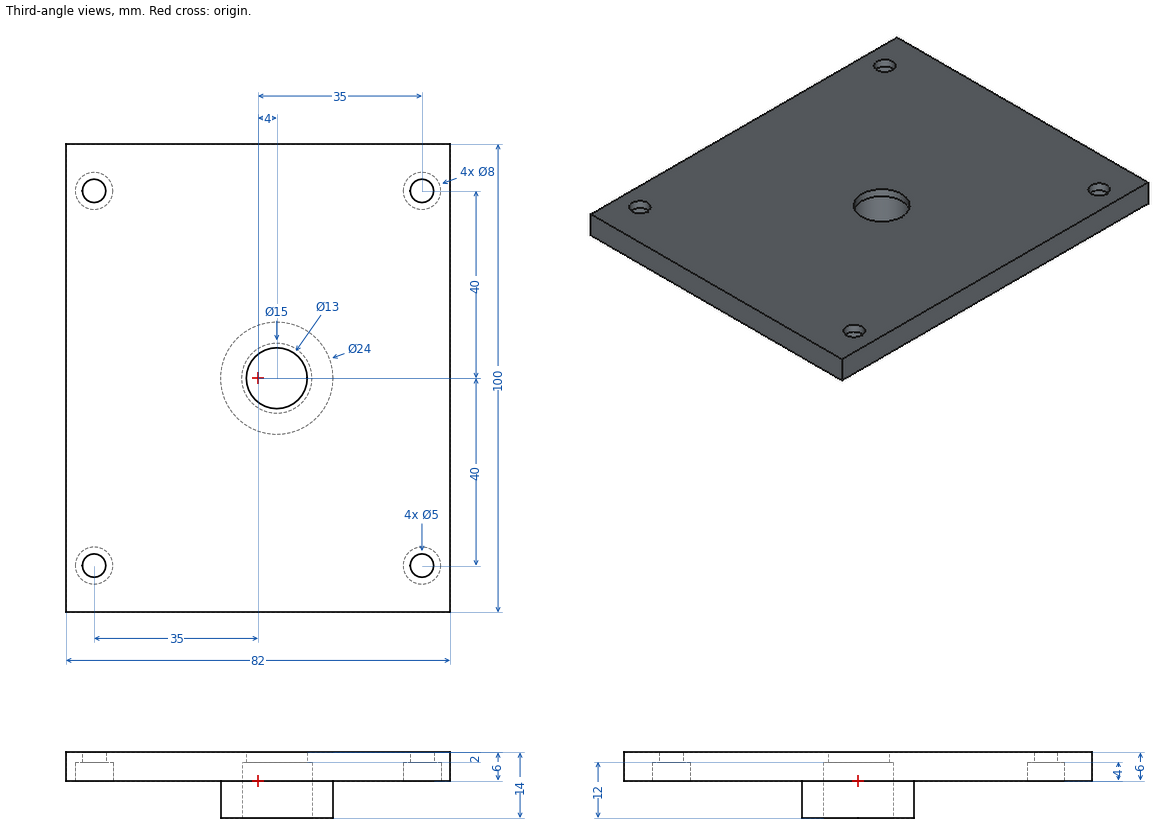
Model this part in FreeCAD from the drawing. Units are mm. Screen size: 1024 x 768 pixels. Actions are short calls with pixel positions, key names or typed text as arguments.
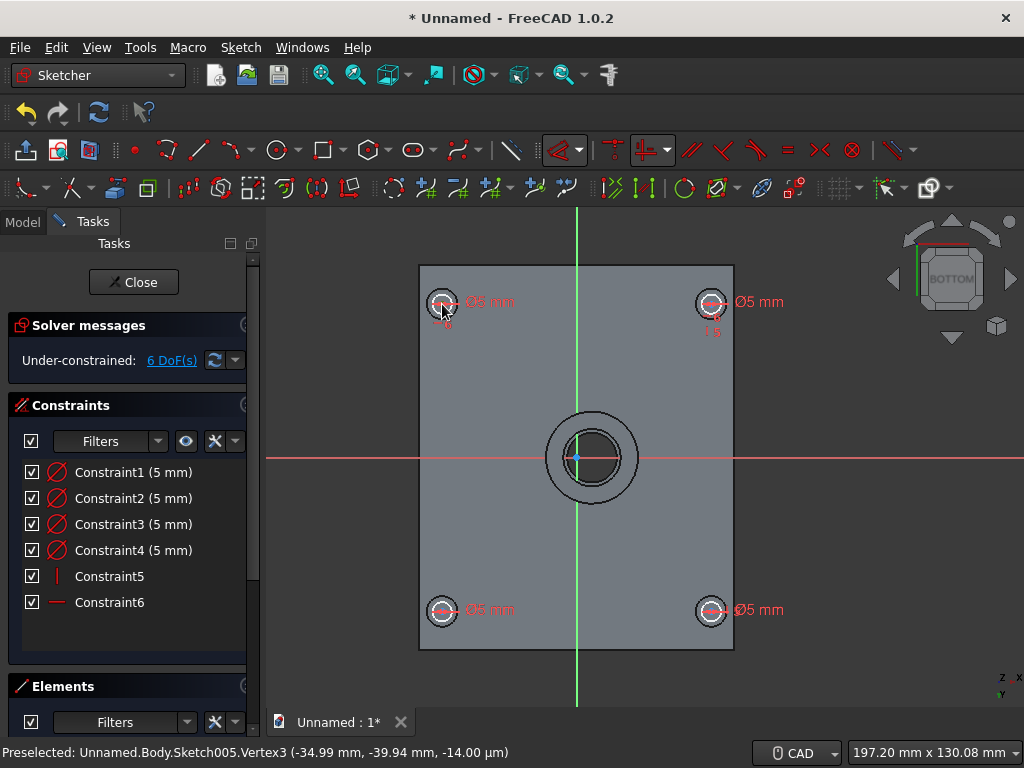
click(442, 612)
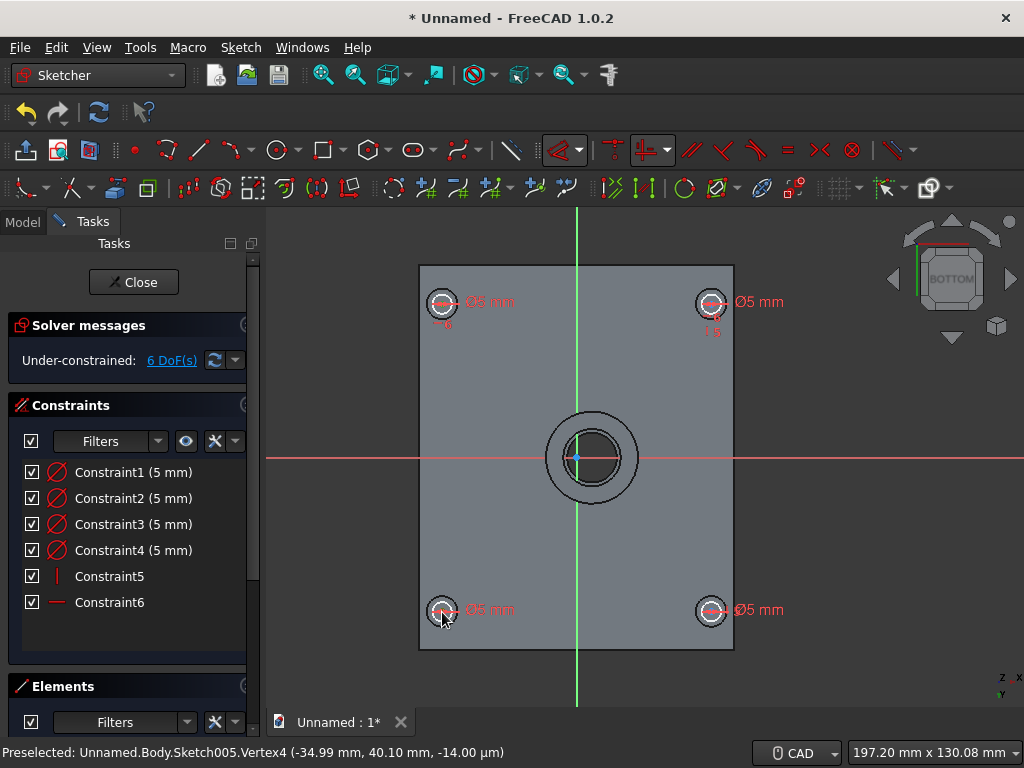
click(670, 150)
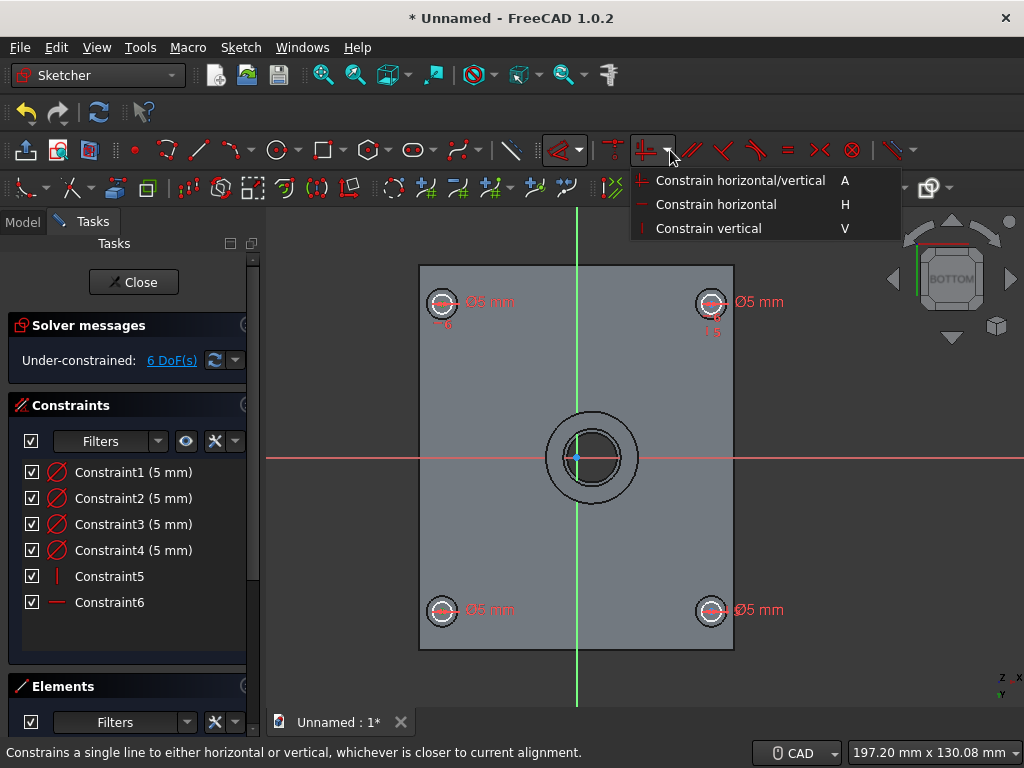
click(766, 228)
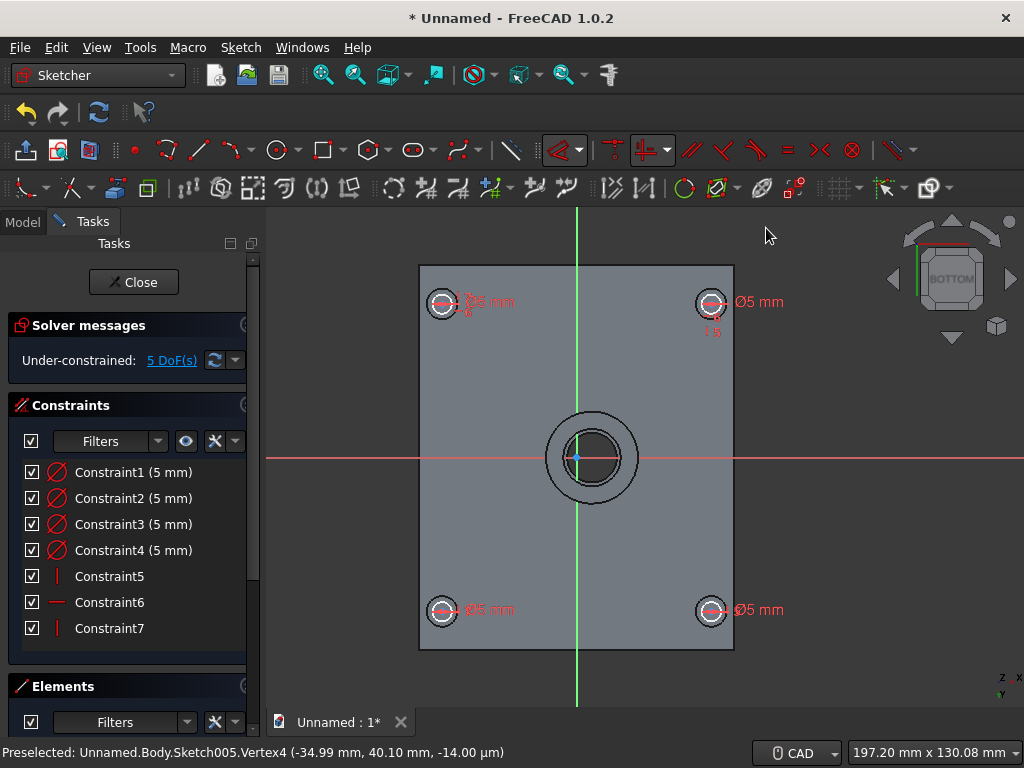
click(711, 612)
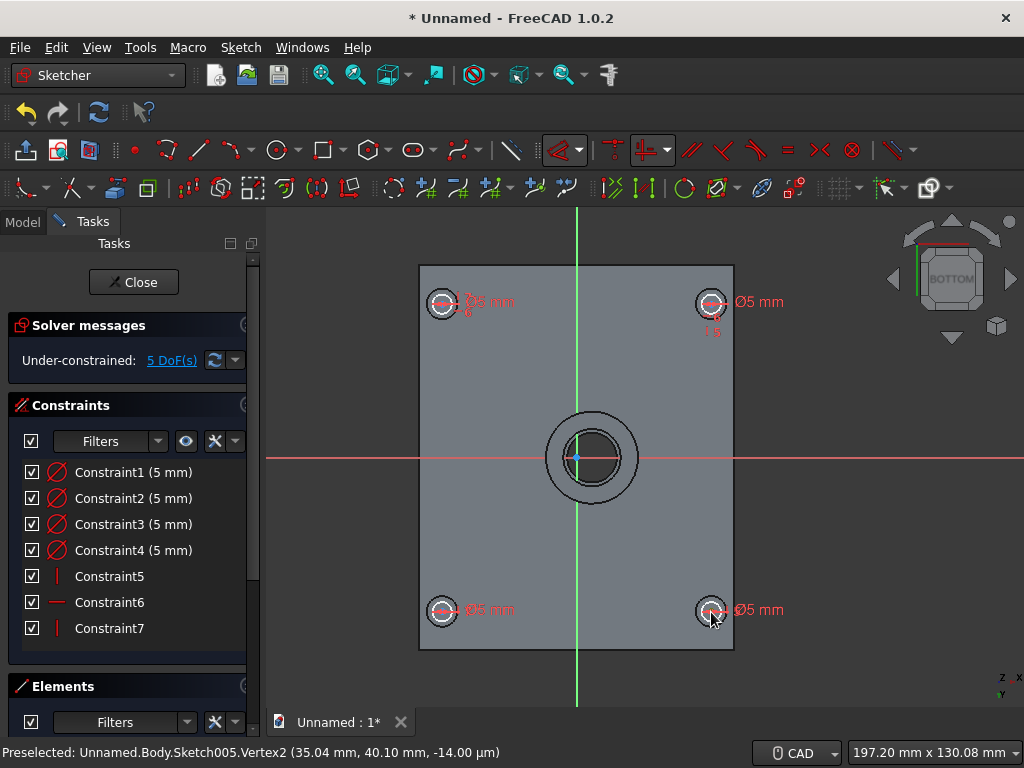
click(442, 612)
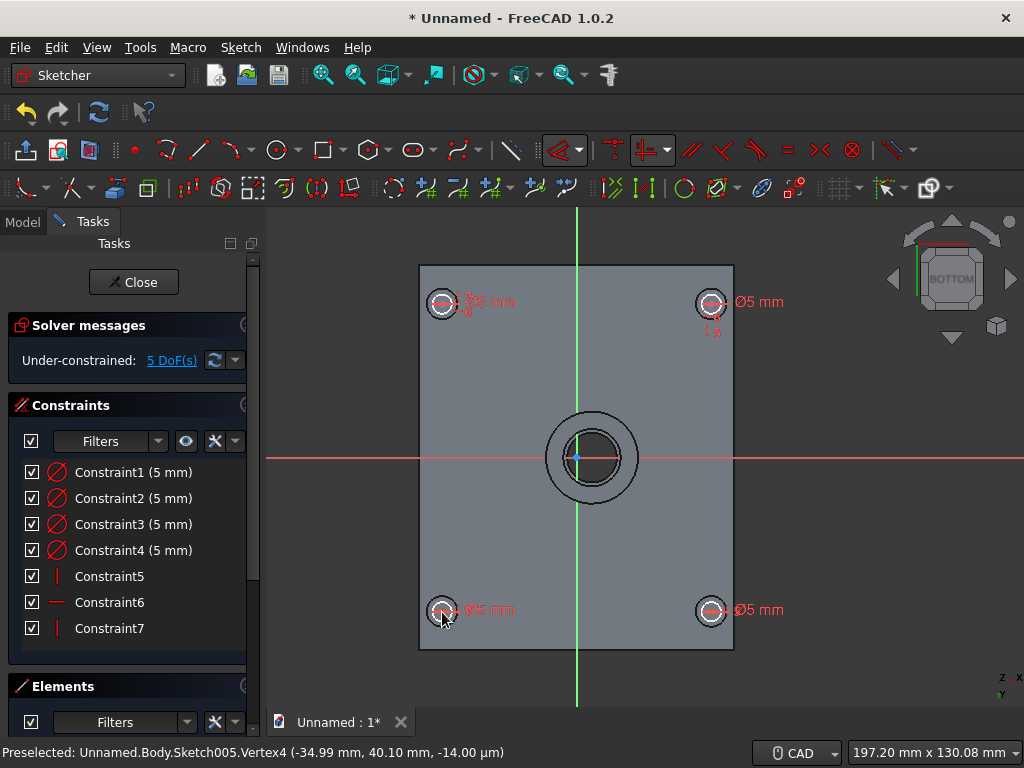
key(h)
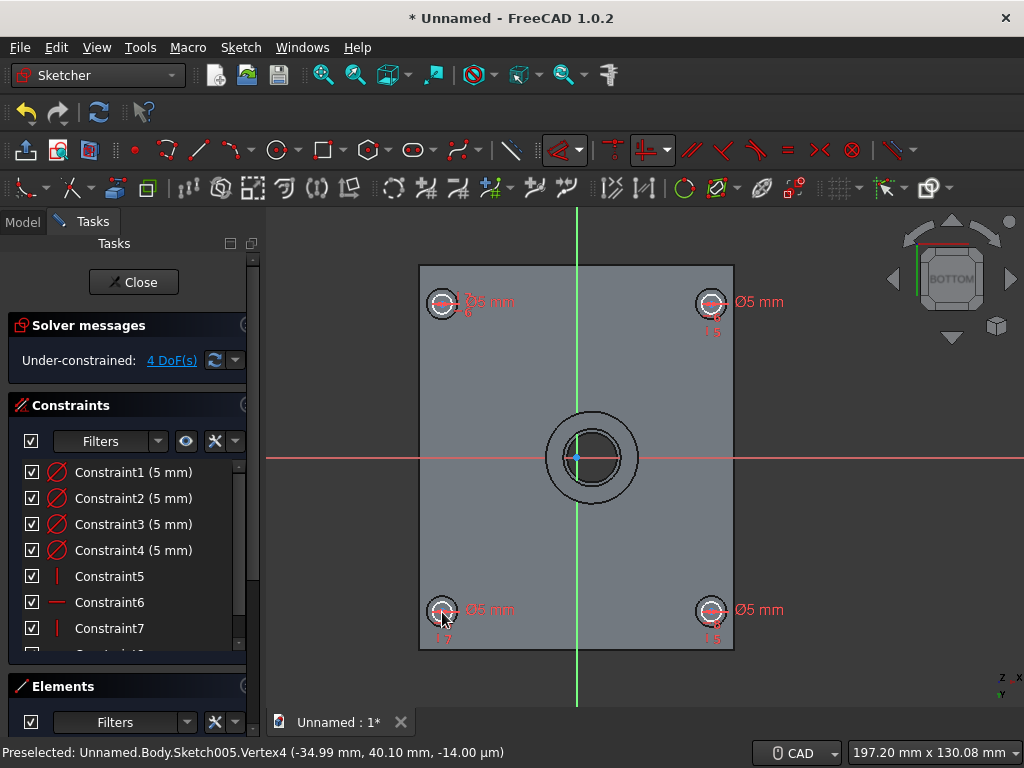
click(711, 304)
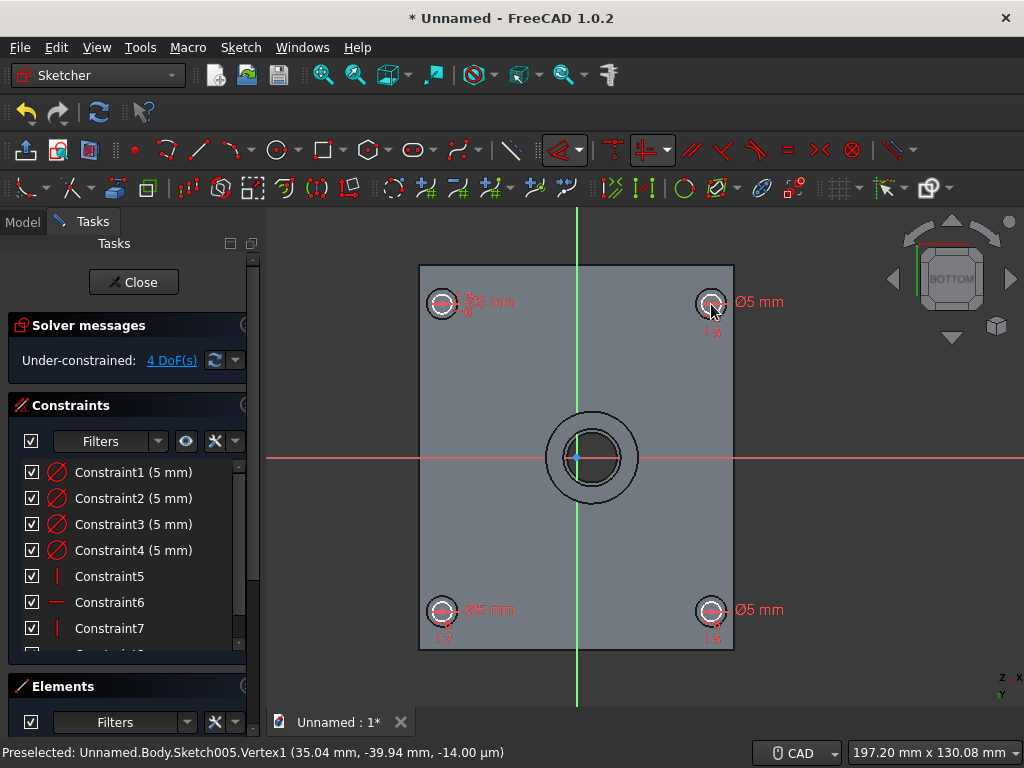
click(582, 150)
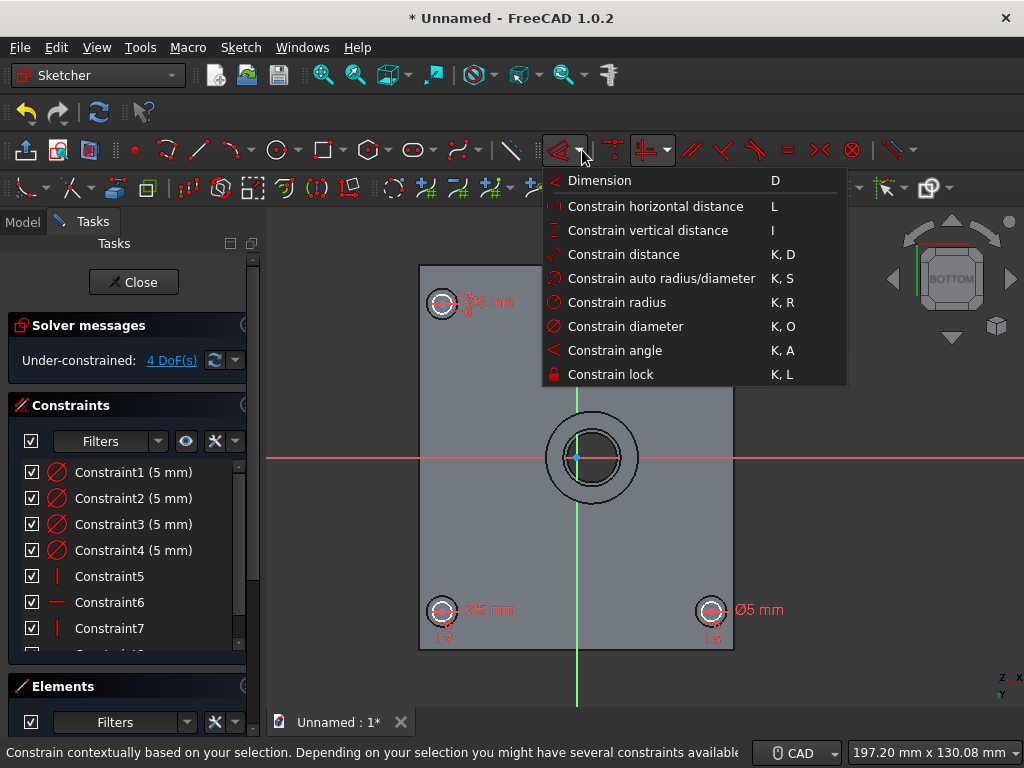
click(695, 206)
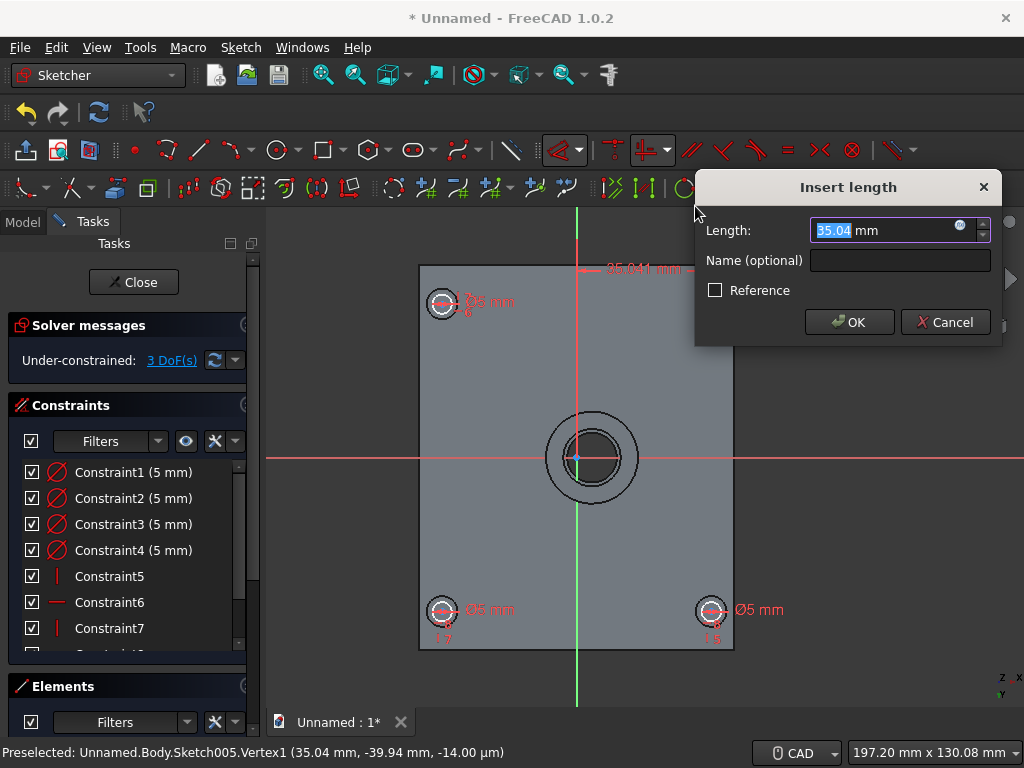
text(35)
key(Return)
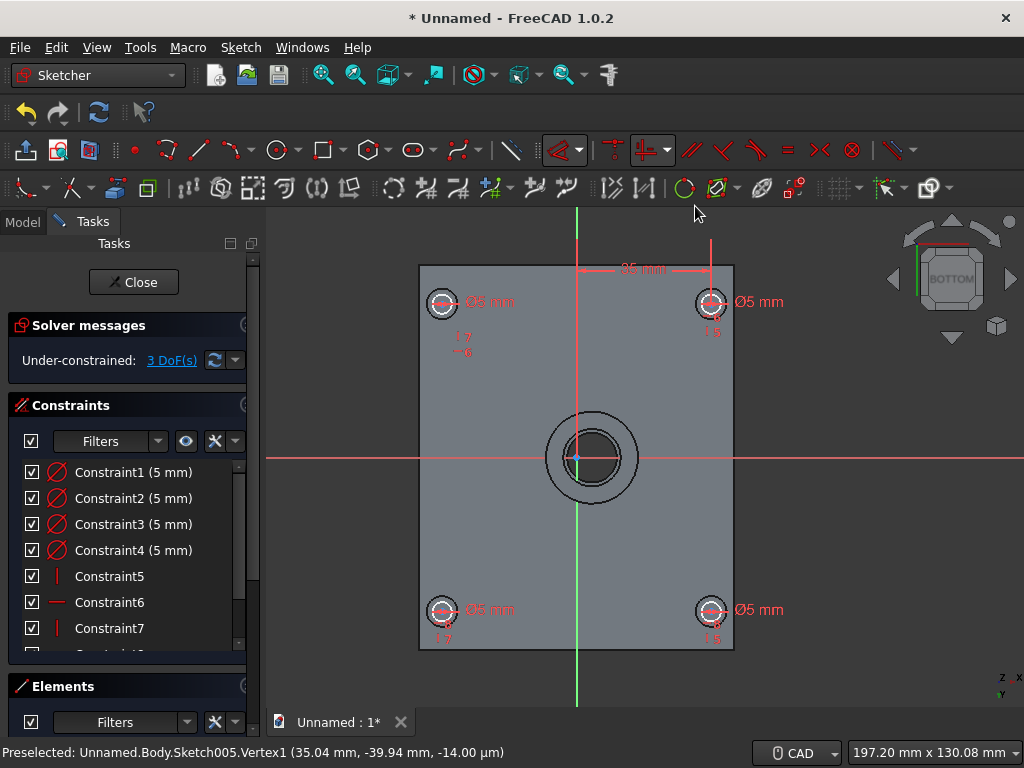
click(711, 304)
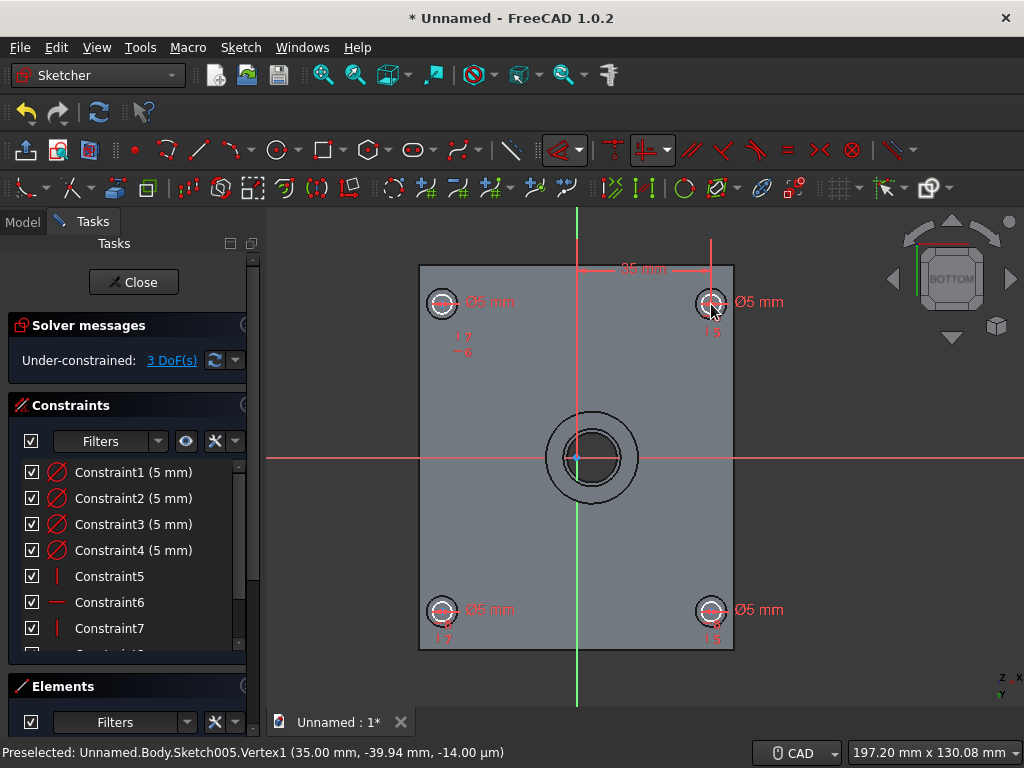
click(582, 150)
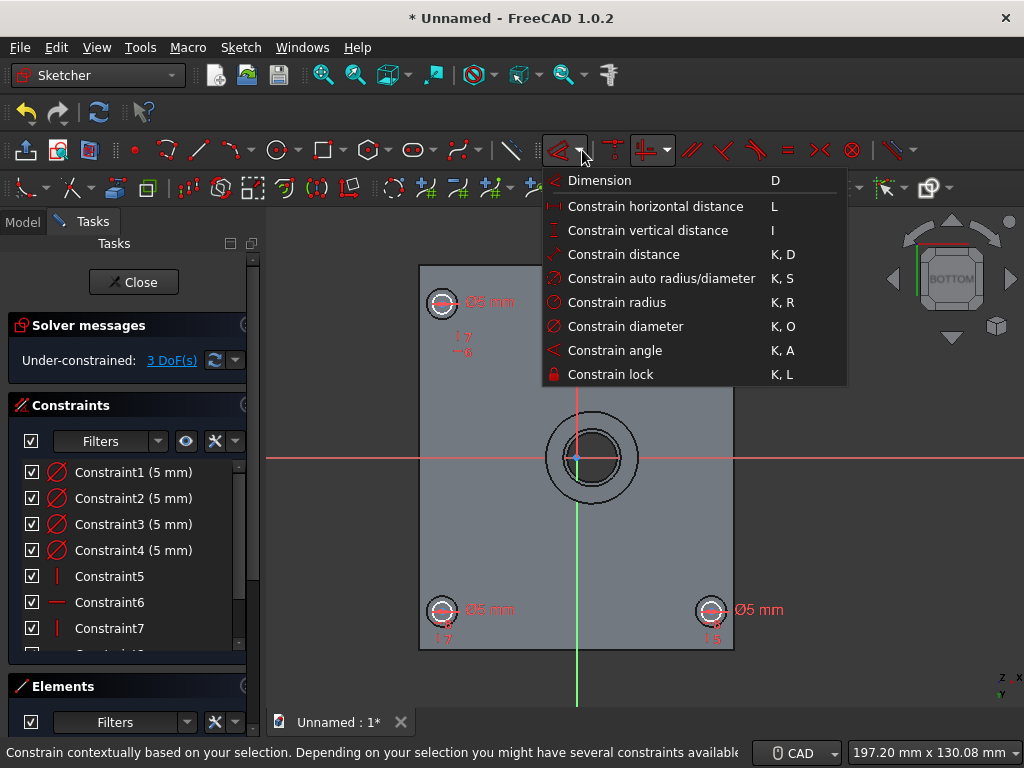
click(695, 230)